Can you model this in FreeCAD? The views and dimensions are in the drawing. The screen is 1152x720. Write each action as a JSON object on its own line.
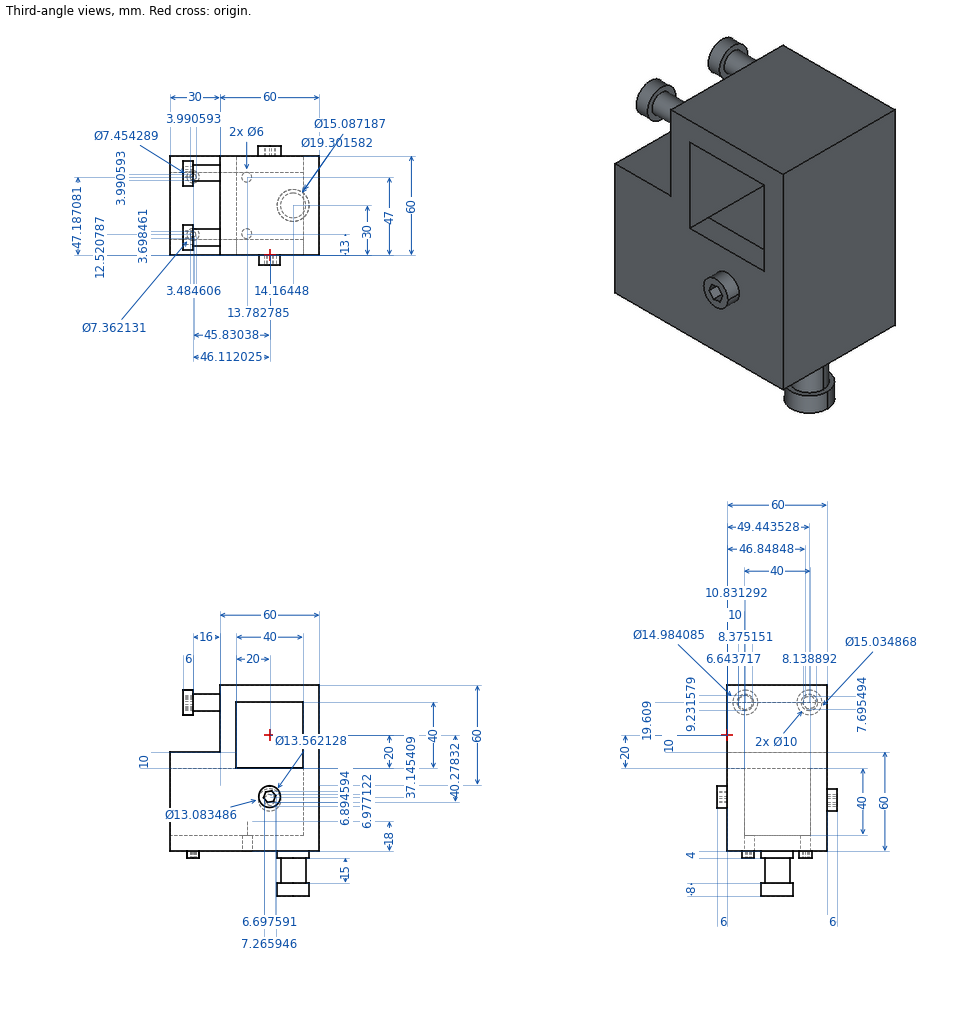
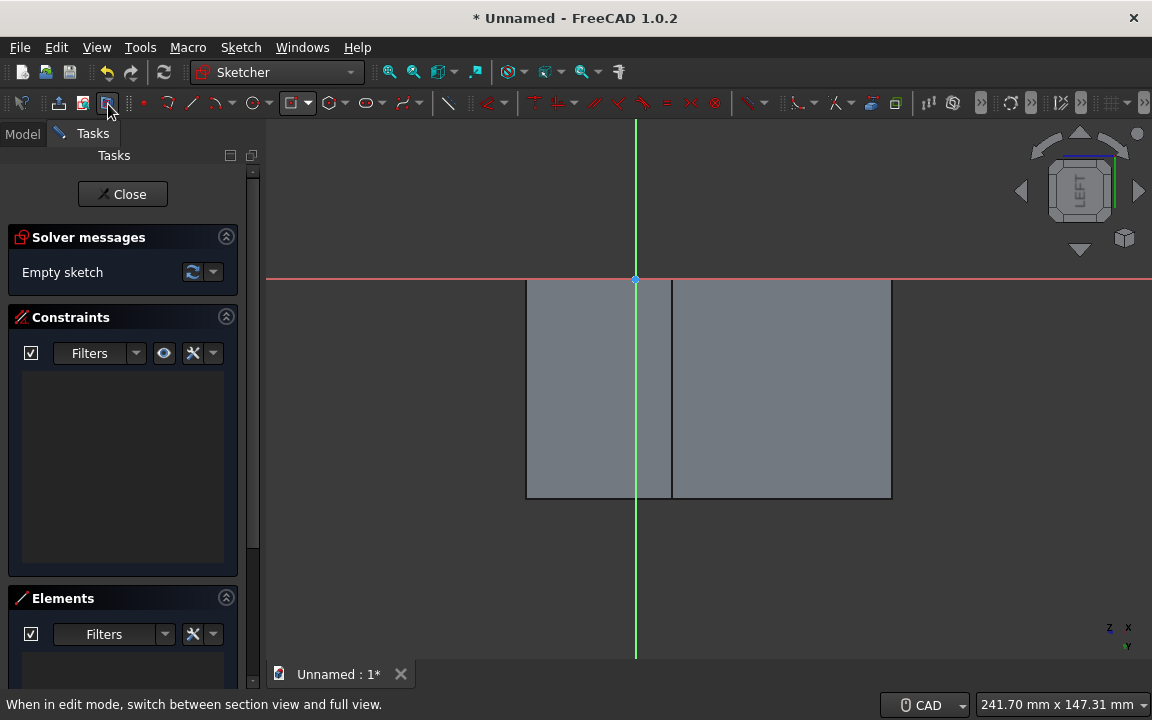
{"action": "scroll", "coordinate": [874, 348], "scroll_direction": "up", "scroll_amount": 3}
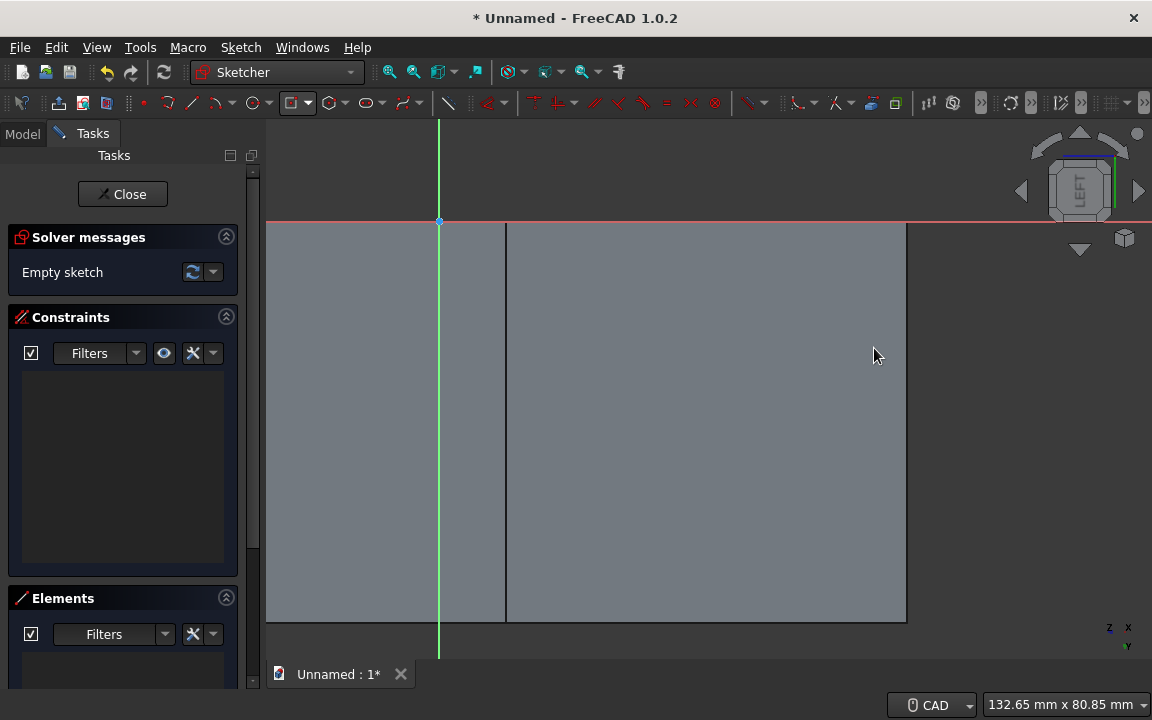
{"action": "key", "text": "g r"}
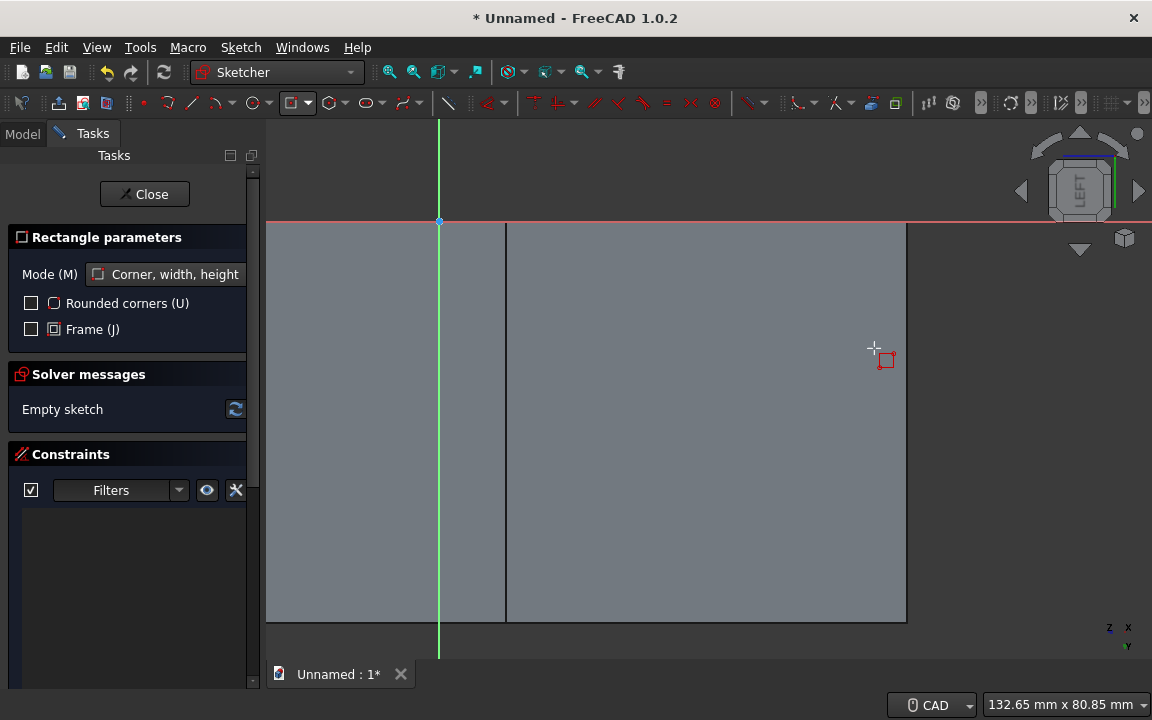
{"action": "left_click", "coordinate": [573, 289]}
{"action": "left_click", "coordinate": [840, 556]}
{"action": "key", "text": "Escape"}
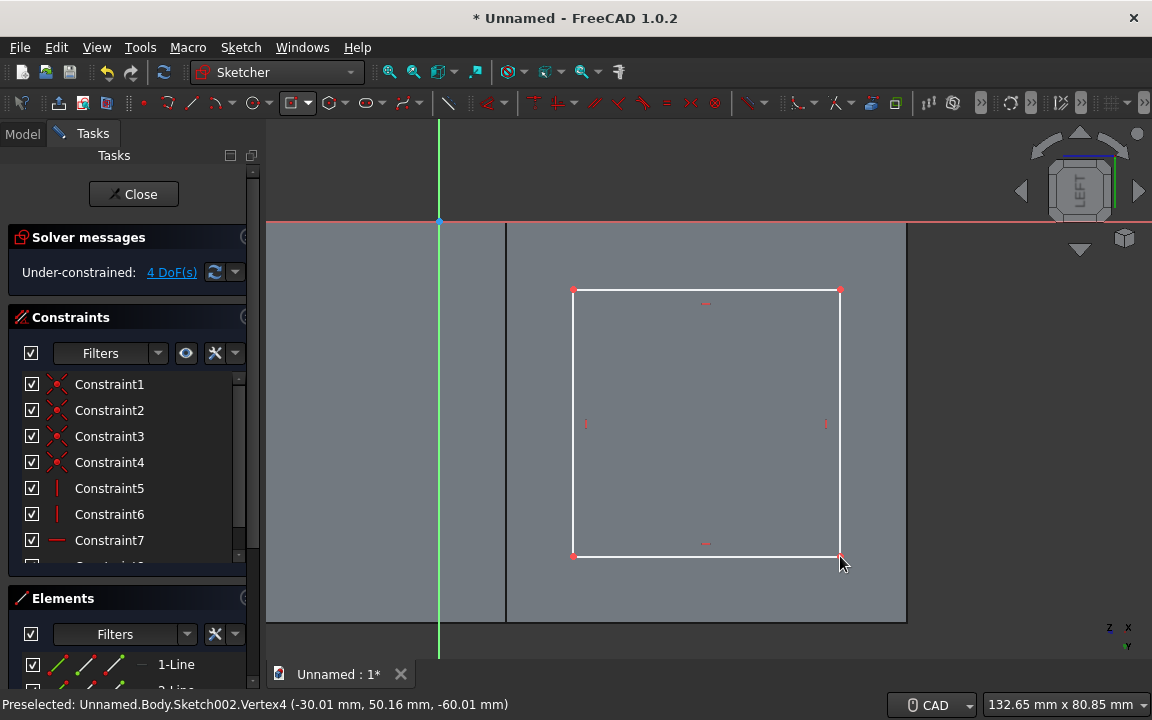
{"action": "left_click", "coordinate": [488, 104]}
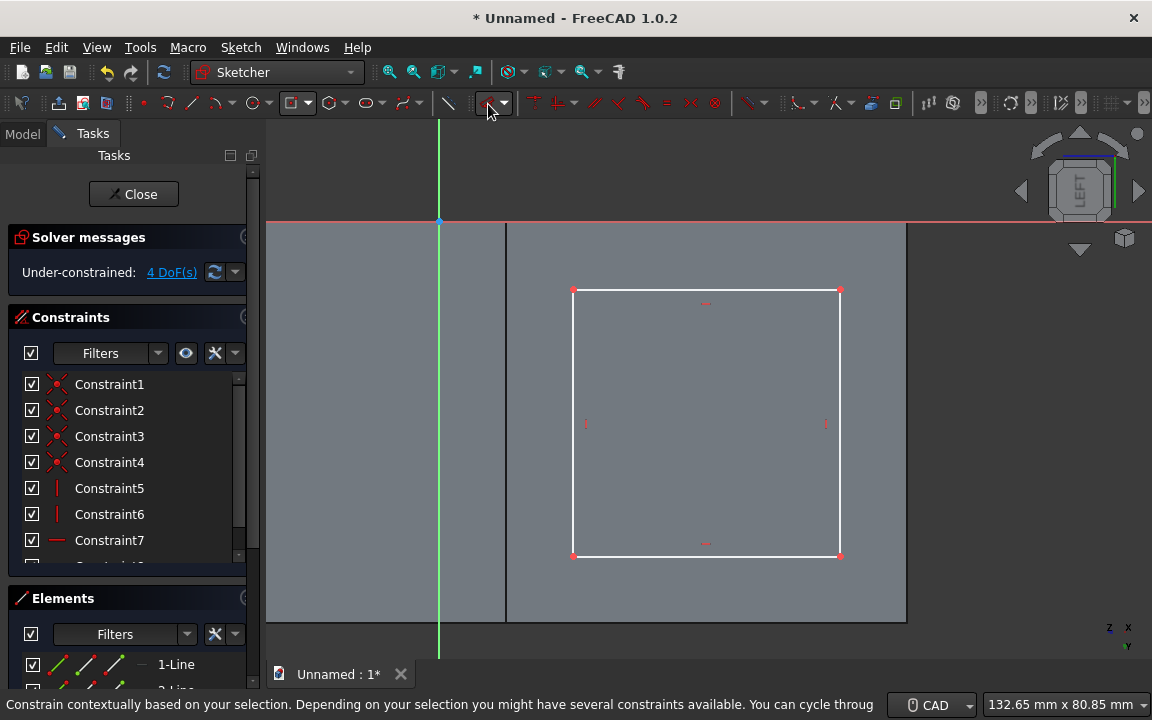
{"action": "left_click", "coordinate": [573, 370]}
{"action": "left_click", "coordinate": [539, 423]}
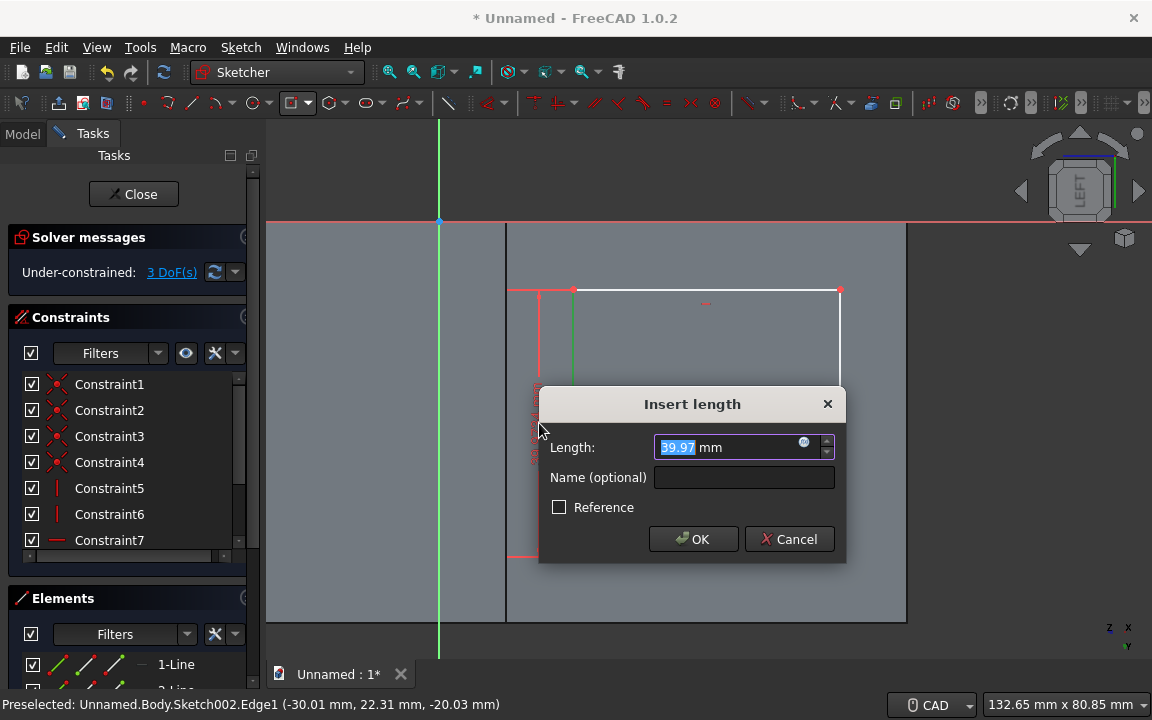
{"action": "type", "text": "40"}
{"action": "key", "text": "Return"}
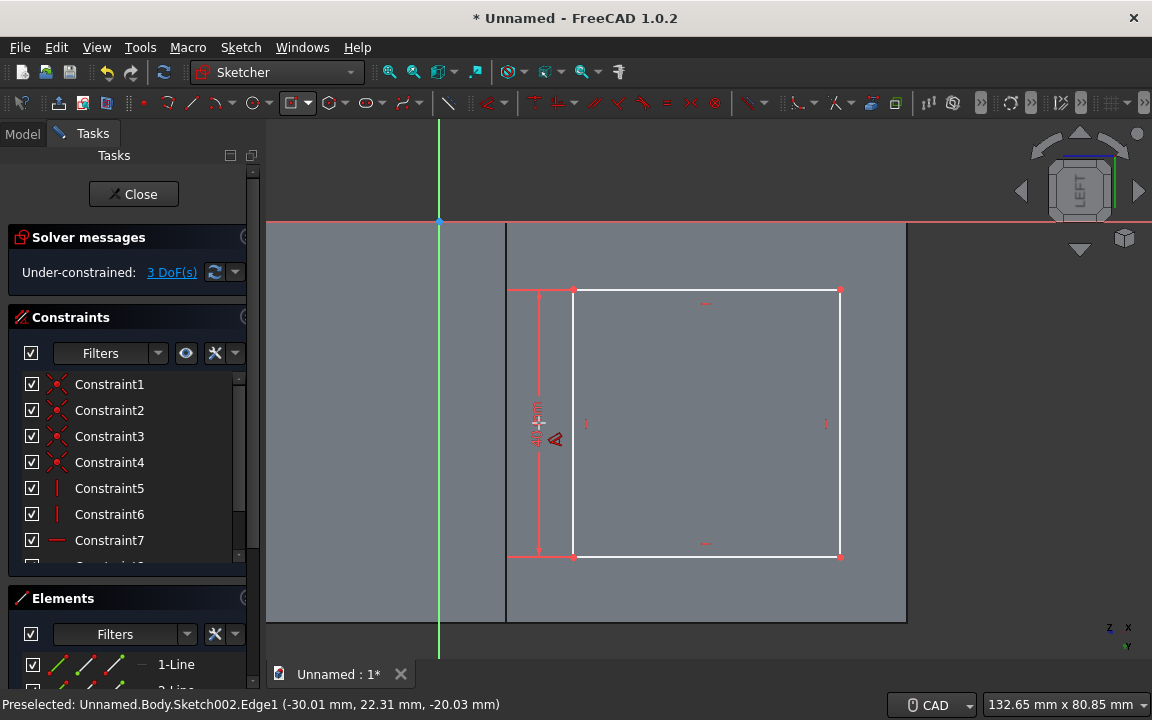
{"action": "left_click", "coordinate": [653, 557]}
{"action": "left_click", "coordinate": [706, 591]}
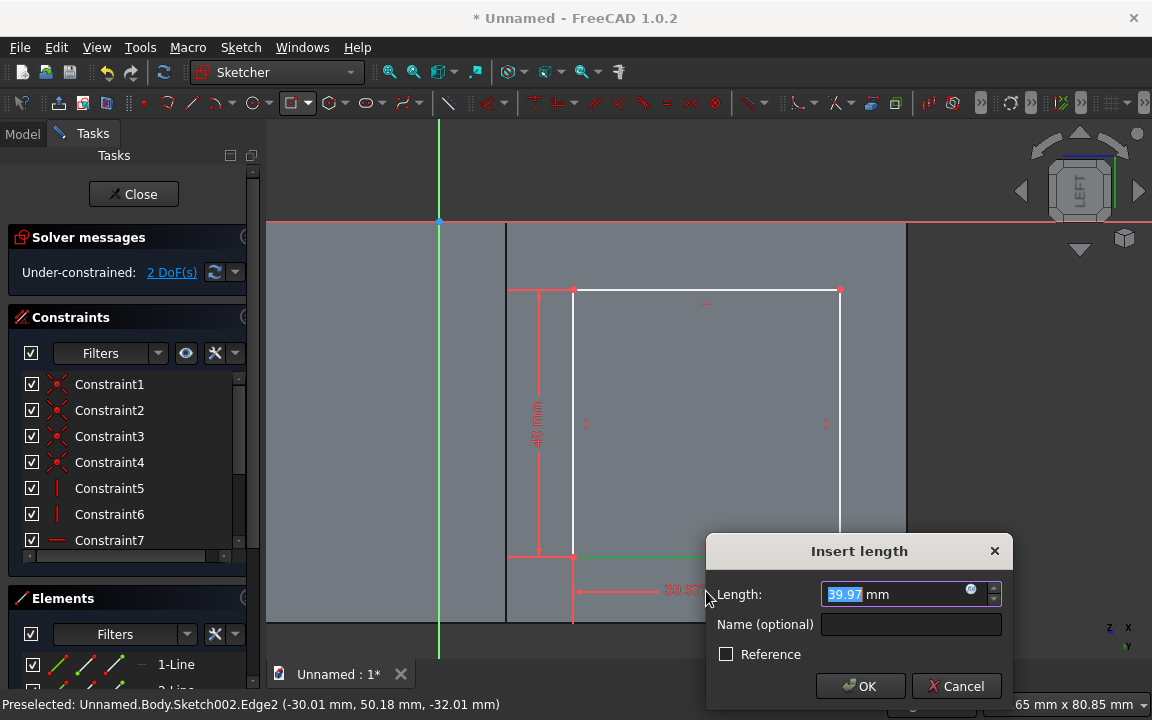
{"action": "type", "text": "40"}
{"action": "key", "text": "Return"}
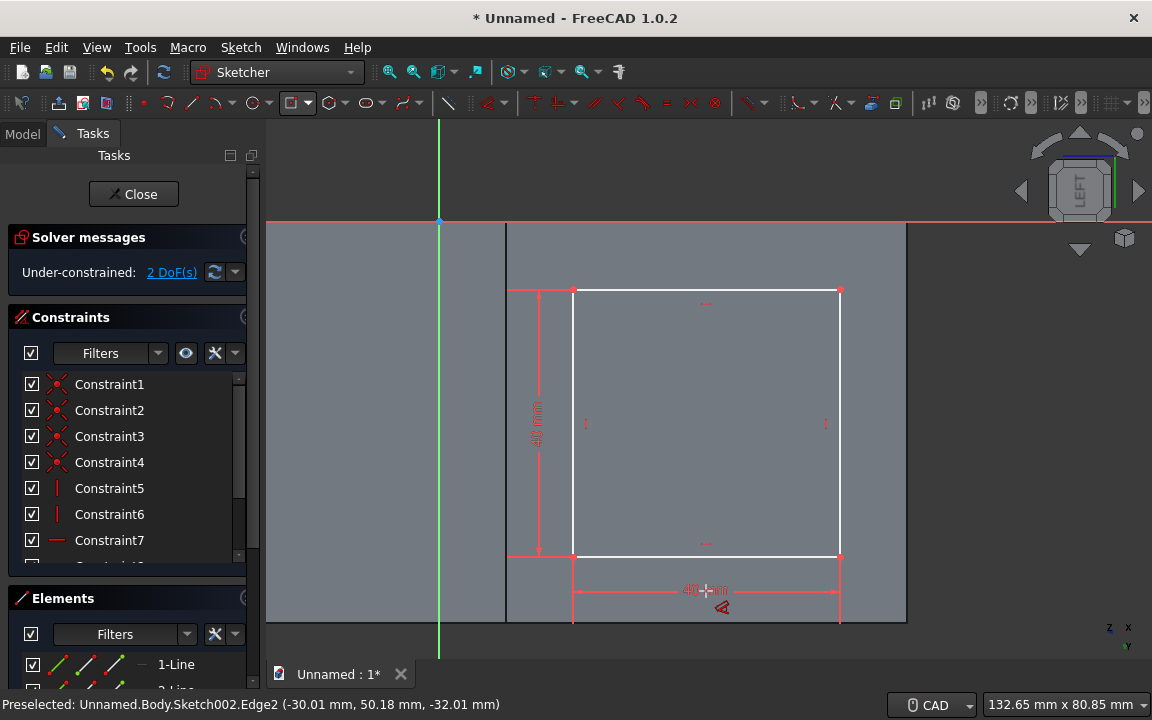
{"action": "left_click", "coordinate": [573, 290]}
{"action": "left_click", "coordinate": [506, 188]}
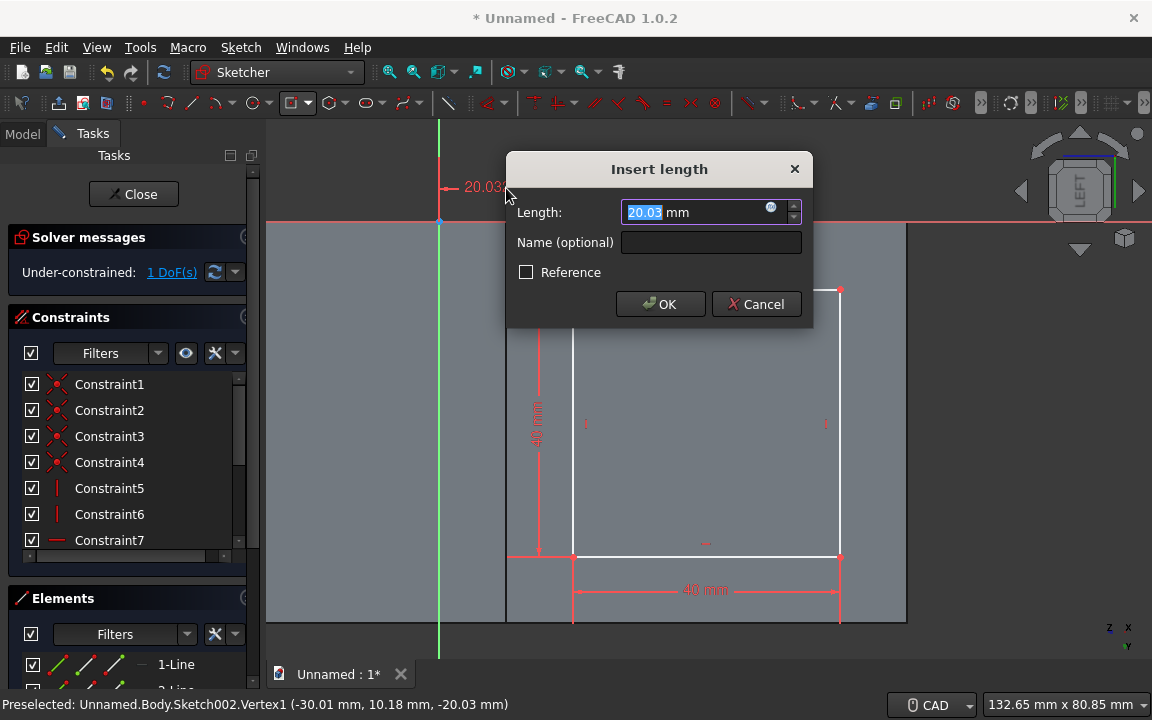
{"action": "type", "text": "20"}
{"action": "key", "text": "Return"}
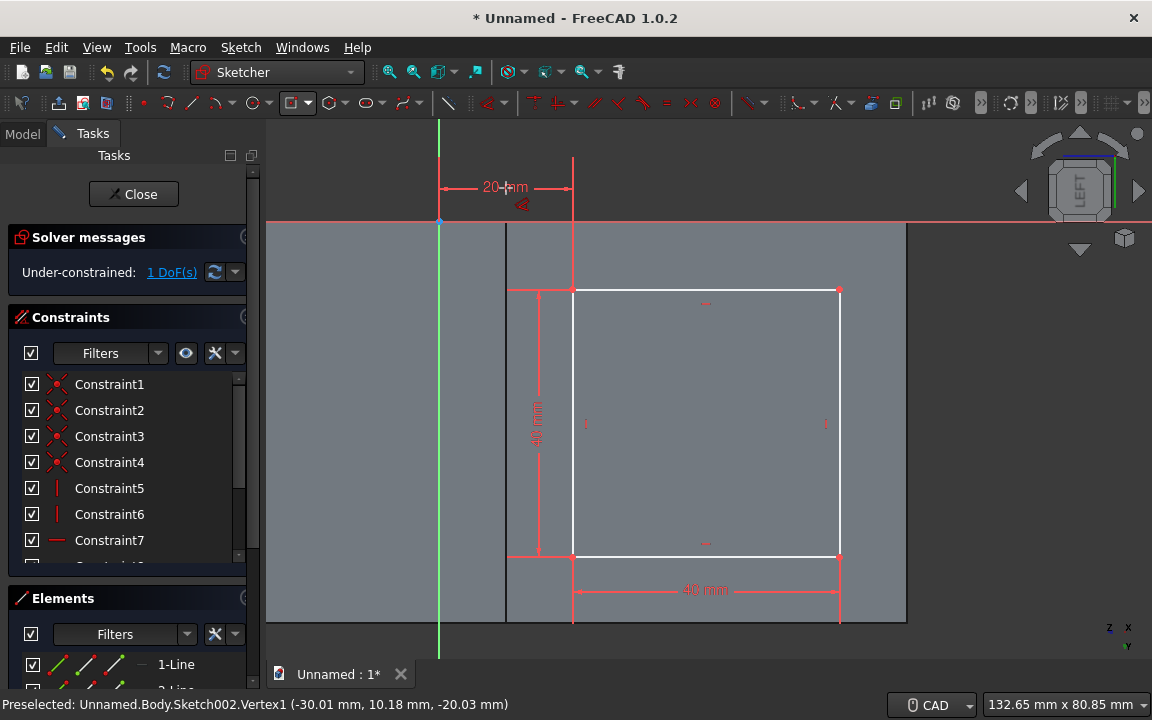
{"action": "left_click", "coordinate": [573, 290]}
{"action": "left_click", "coordinate": [405, 256]}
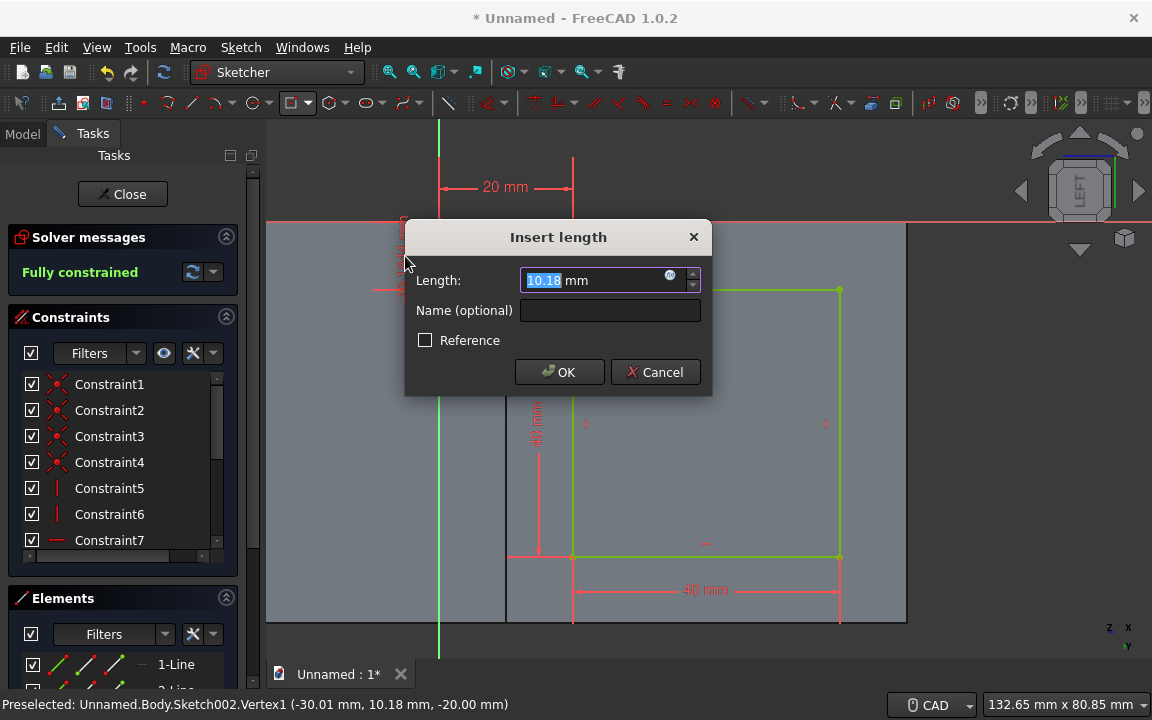
{"action": "type", "text": "10"}
{"action": "key", "text": "Return"}
{"action": "key", "text": "Escape"}